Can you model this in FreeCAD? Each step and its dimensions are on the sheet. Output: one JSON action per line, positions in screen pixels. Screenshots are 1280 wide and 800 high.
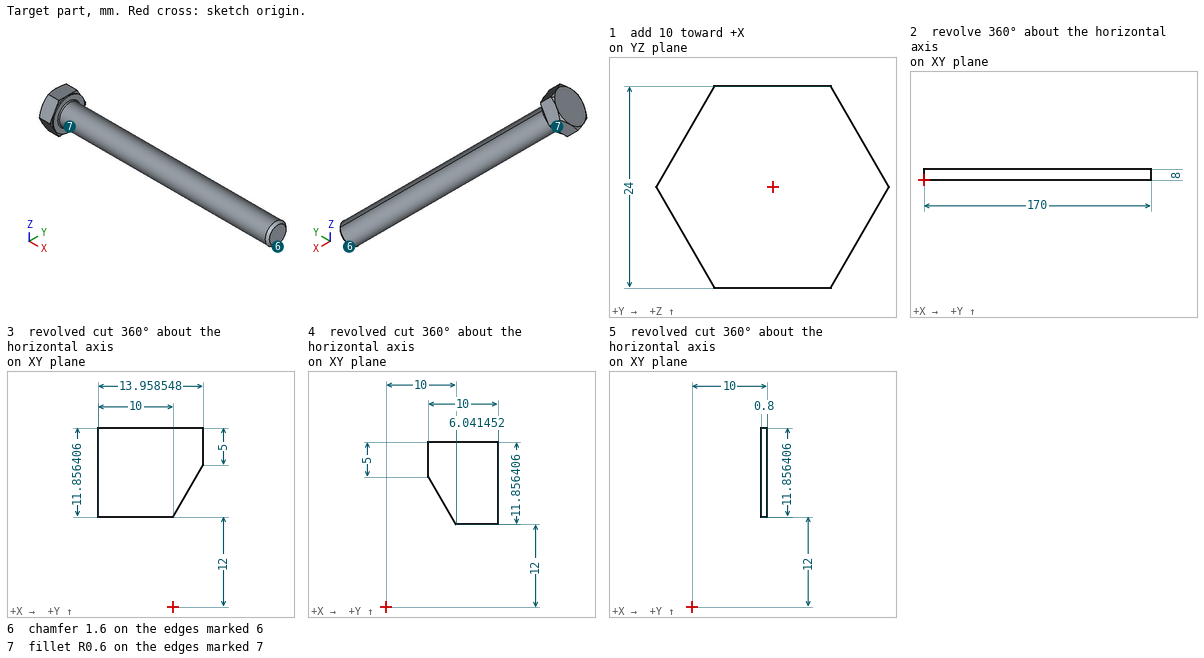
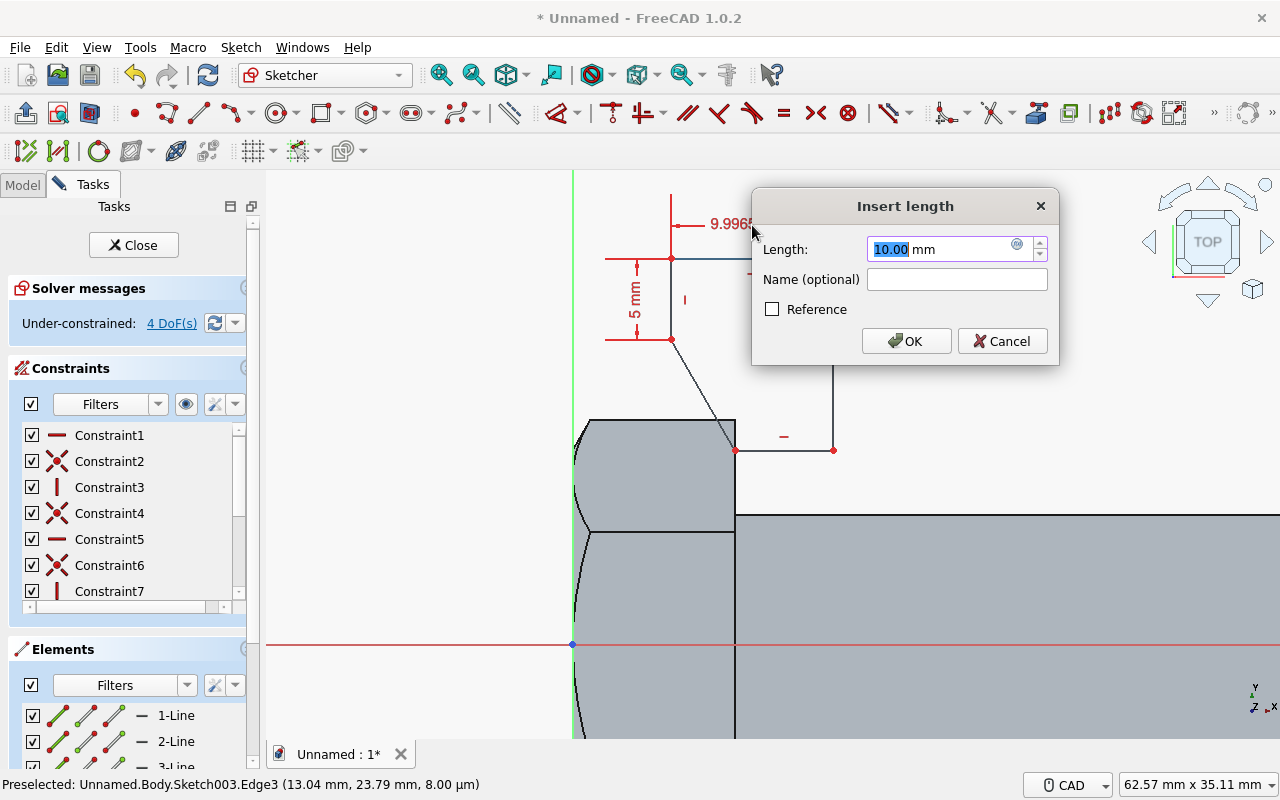
{"action": "type", "text": "10"}
{"action": "key", "text": "Return"}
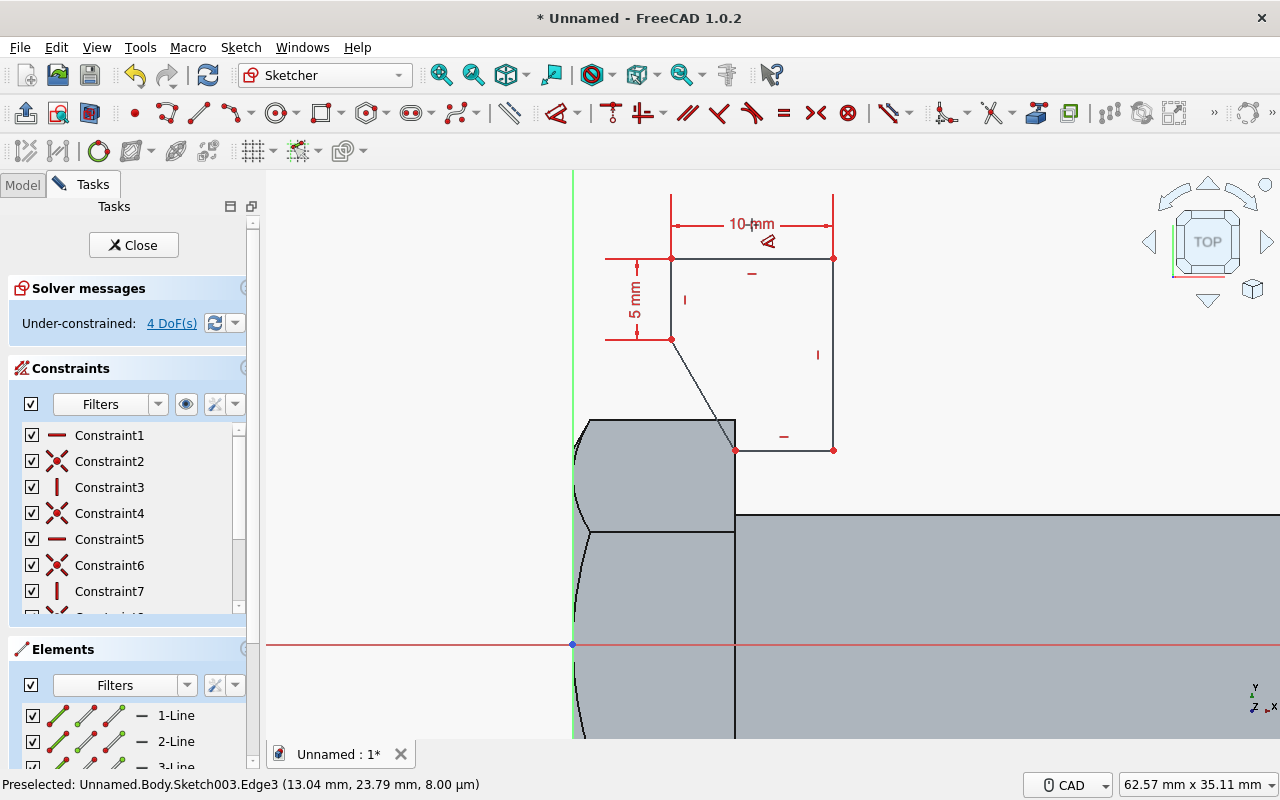
{"action": "left_click", "coordinate": [735, 451]}
{"action": "left_click", "coordinate": [654, 679]}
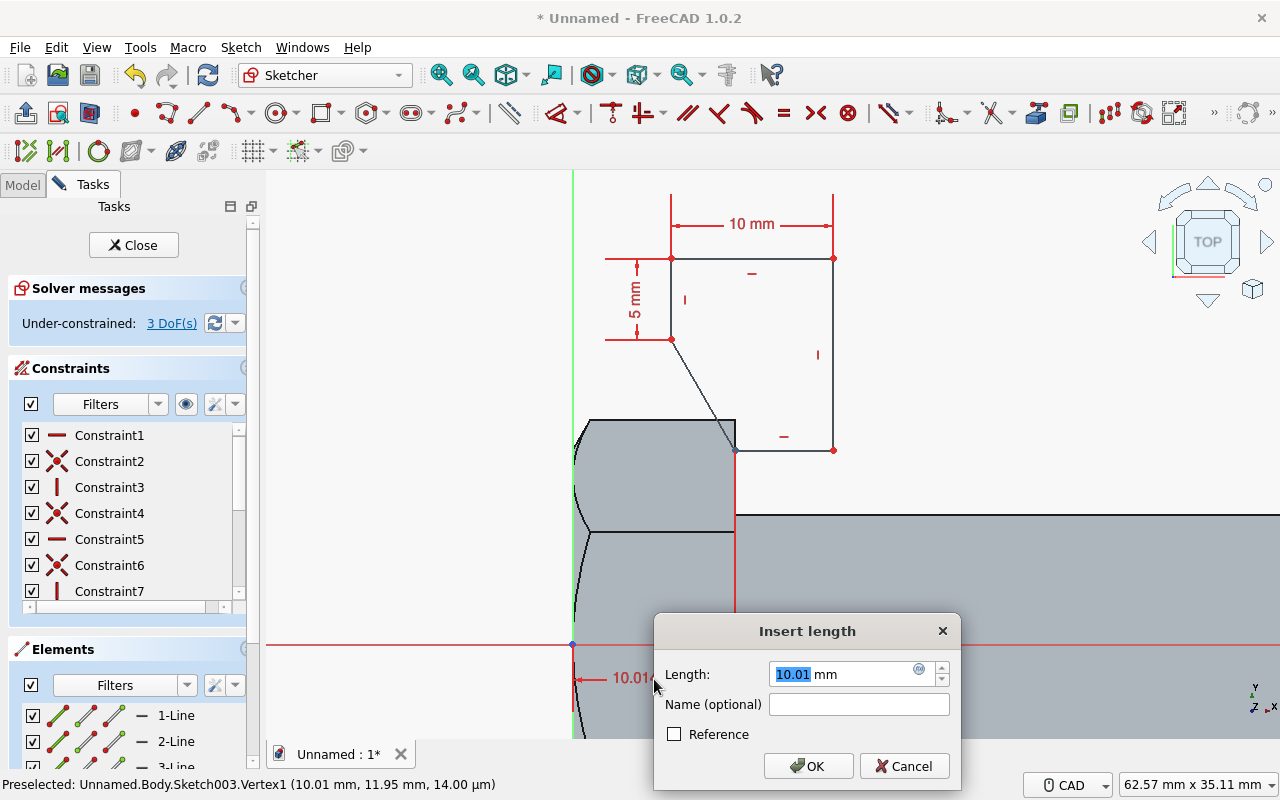
{"action": "type", "text": "10"}
{"action": "key", "text": "Return"}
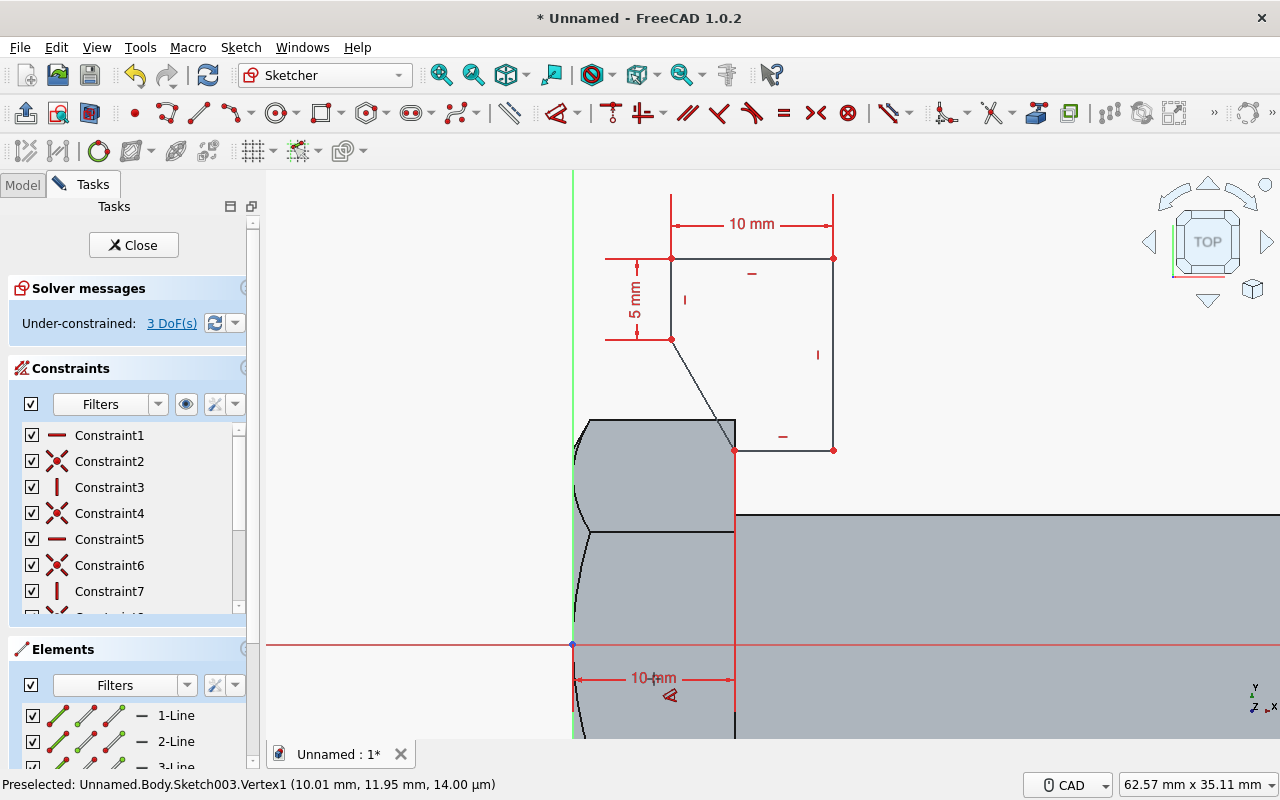
{"action": "left_click", "coordinate": [735, 451]}
{"action": "left_click", "coordinate": [539, 548]}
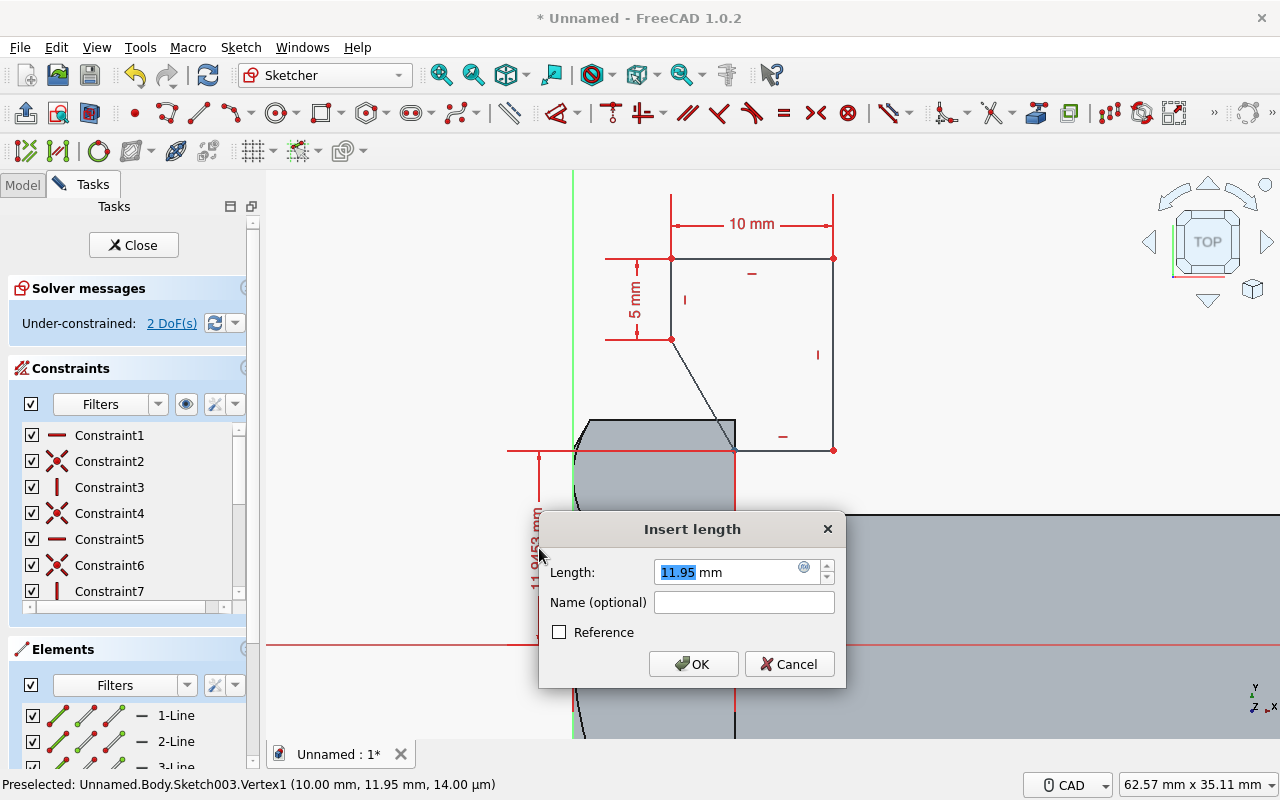
{"action": "type", "text": "12"}
{"action": "key", "text": "Return"}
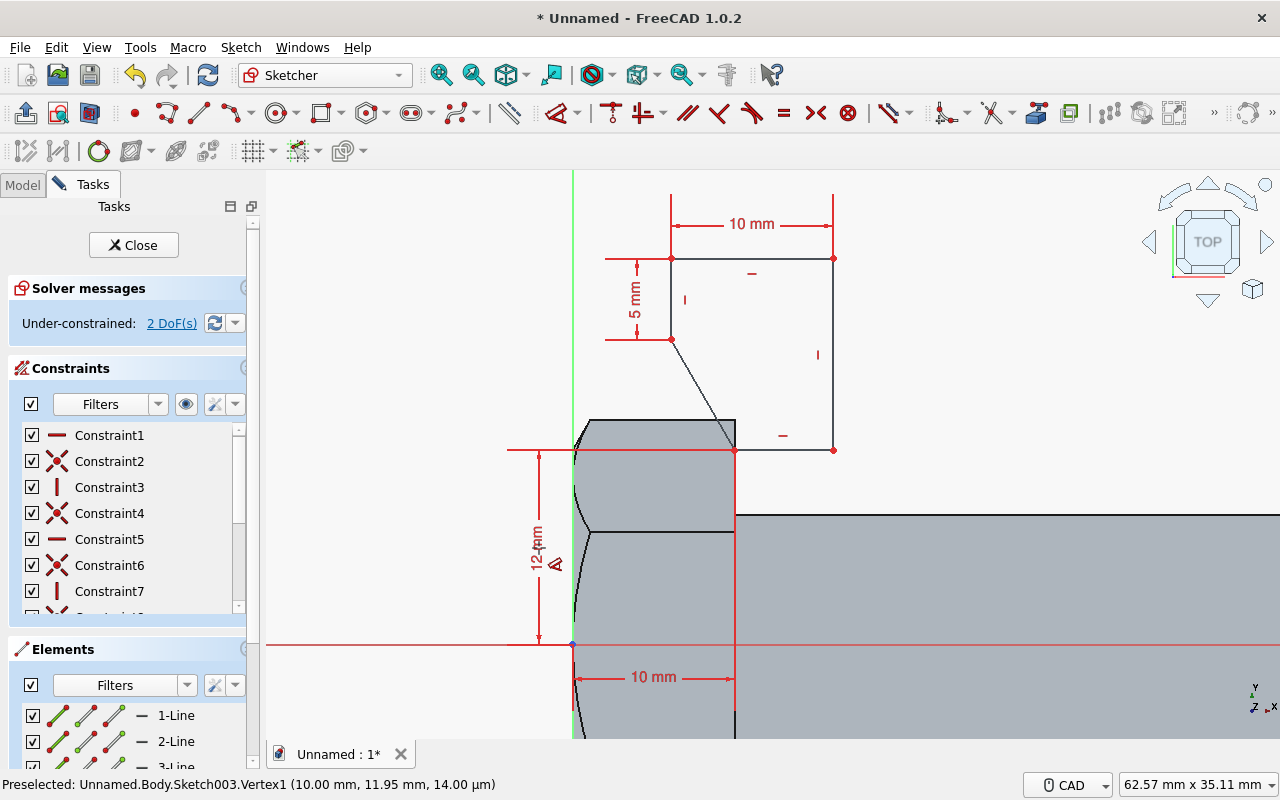
{"action": "left_click", "coordinate": [764, 450]}
{"action": "left_click", "coordinate": [784, 416]}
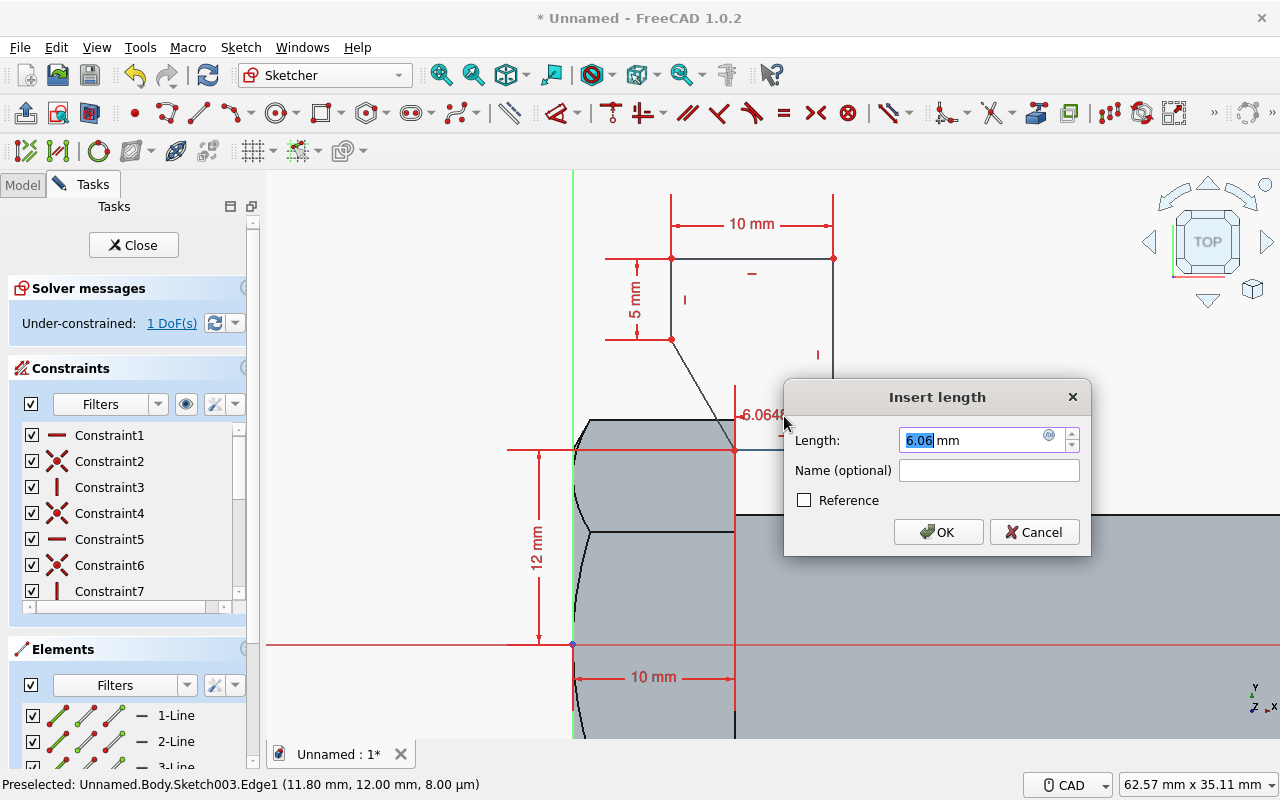
{"action": "type", "text": "6.041452"}
{"action": "key", "text": "Return"}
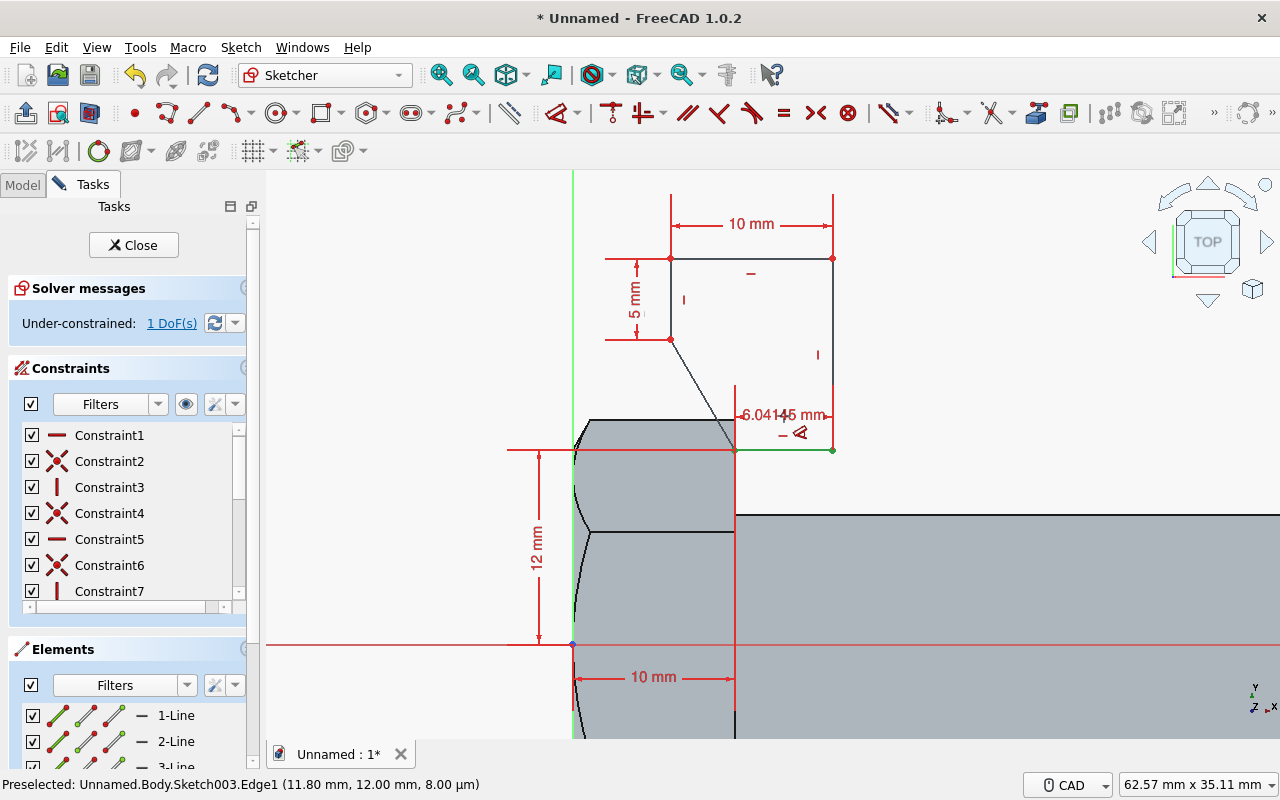
{"action": "left_click", "coordinate": [833, 393]}
{"action": "left_click", "coordinate": [867, 355]}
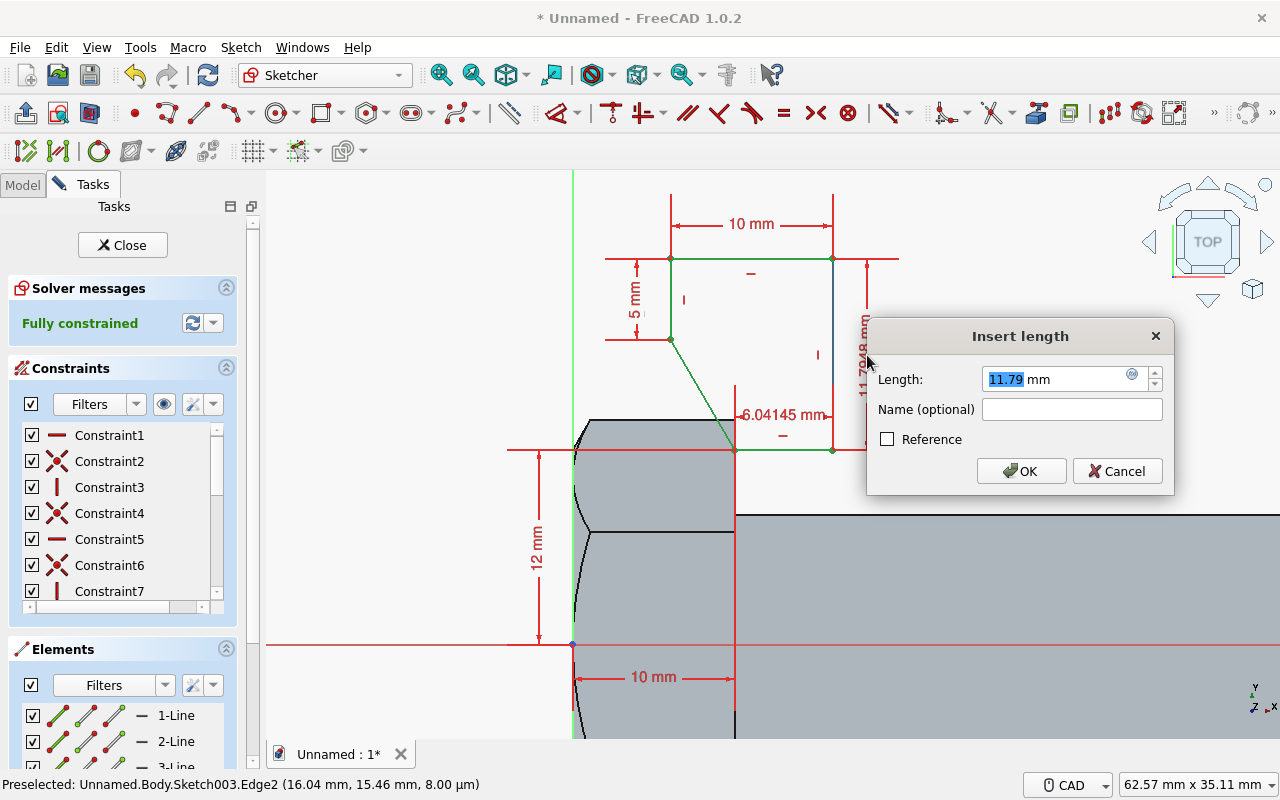
{"action": "type", "text": "11.856406"}
{"action": "key", "text": "Return"}
{"action": "key", "text": "Escape"}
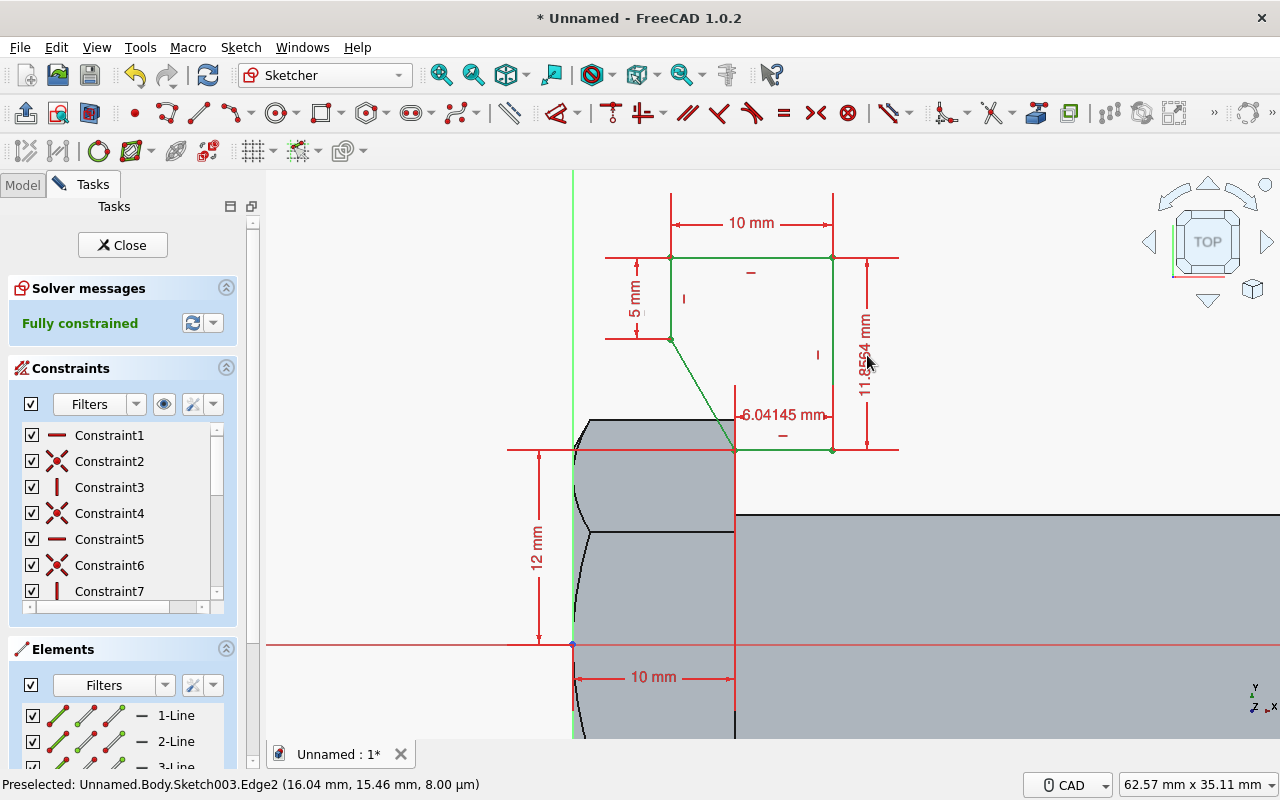
{"action": "left_click", "coordinate": [123, 245]}